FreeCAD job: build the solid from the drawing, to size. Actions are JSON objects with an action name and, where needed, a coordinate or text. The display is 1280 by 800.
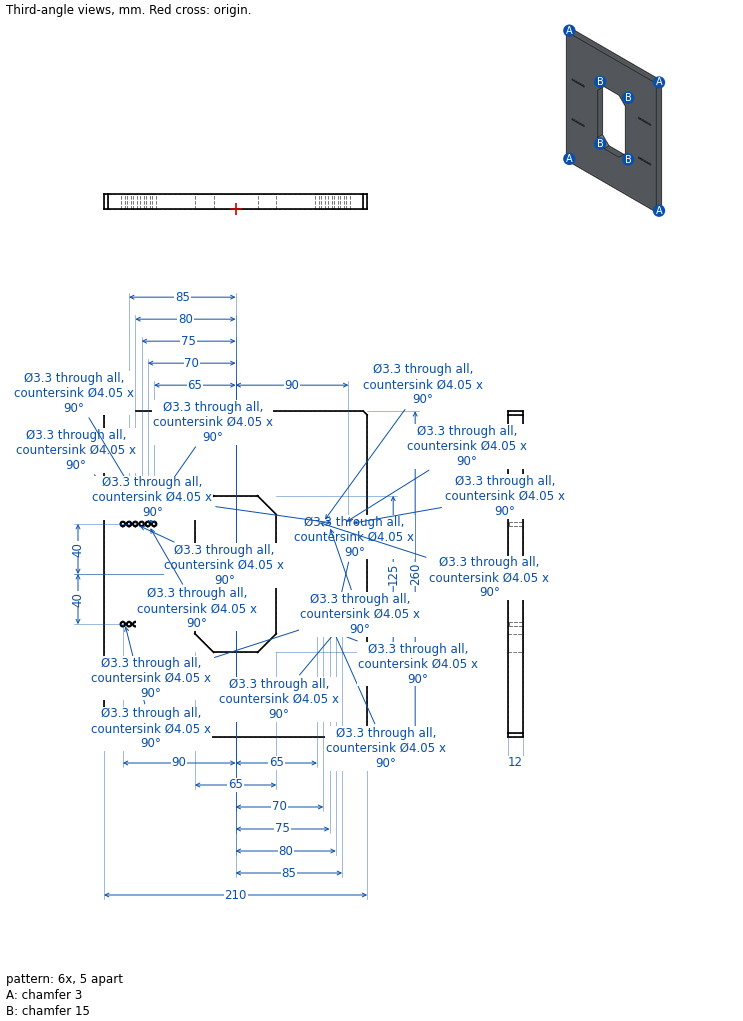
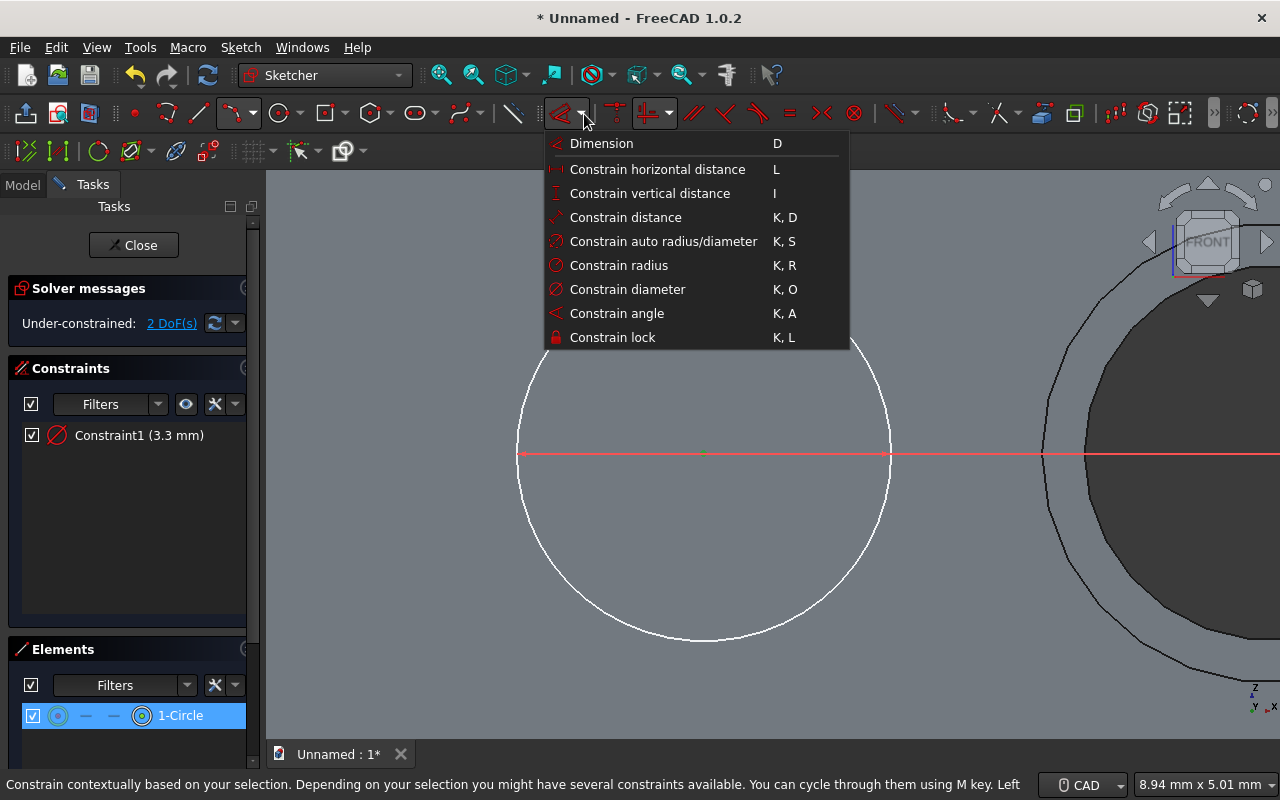
{"action": "left_click", "coordinate": [697, 169]}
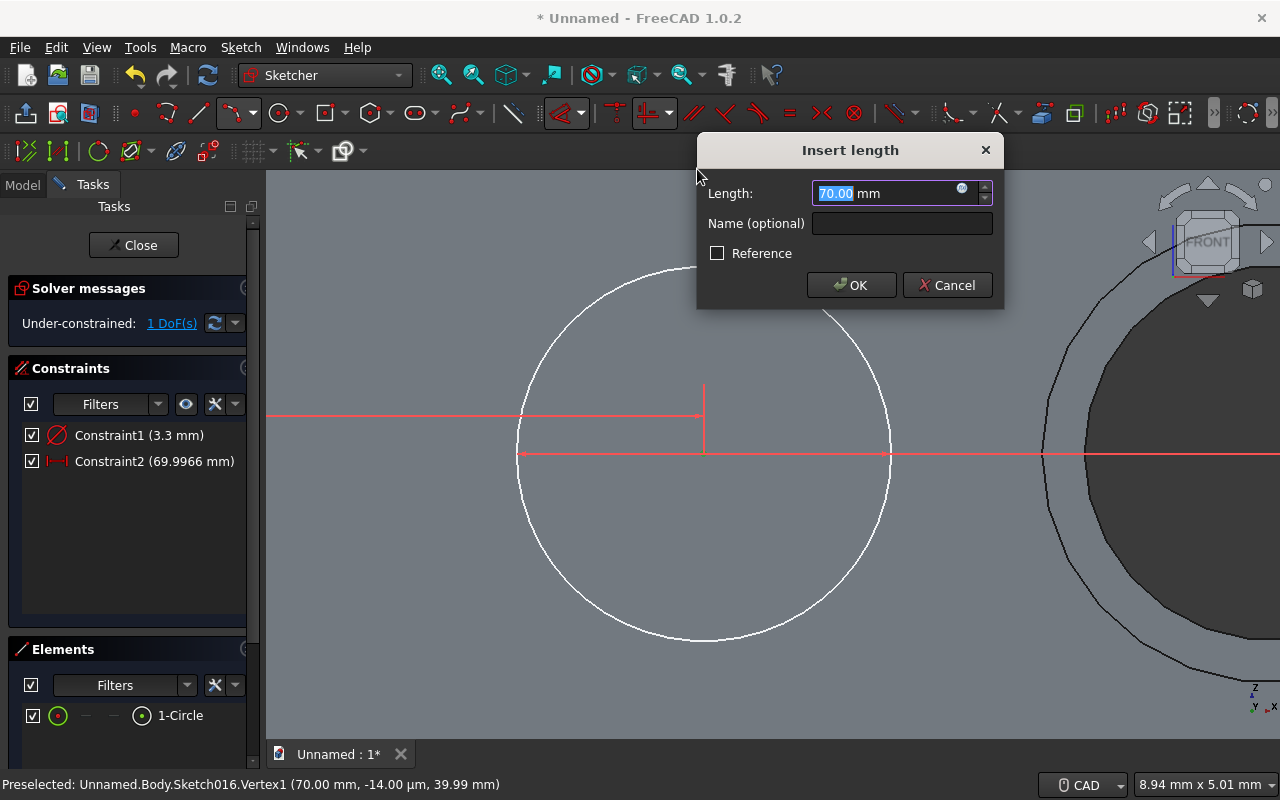
{"action": "type", "text": "70"}
{"action": "key", "text": "Return"}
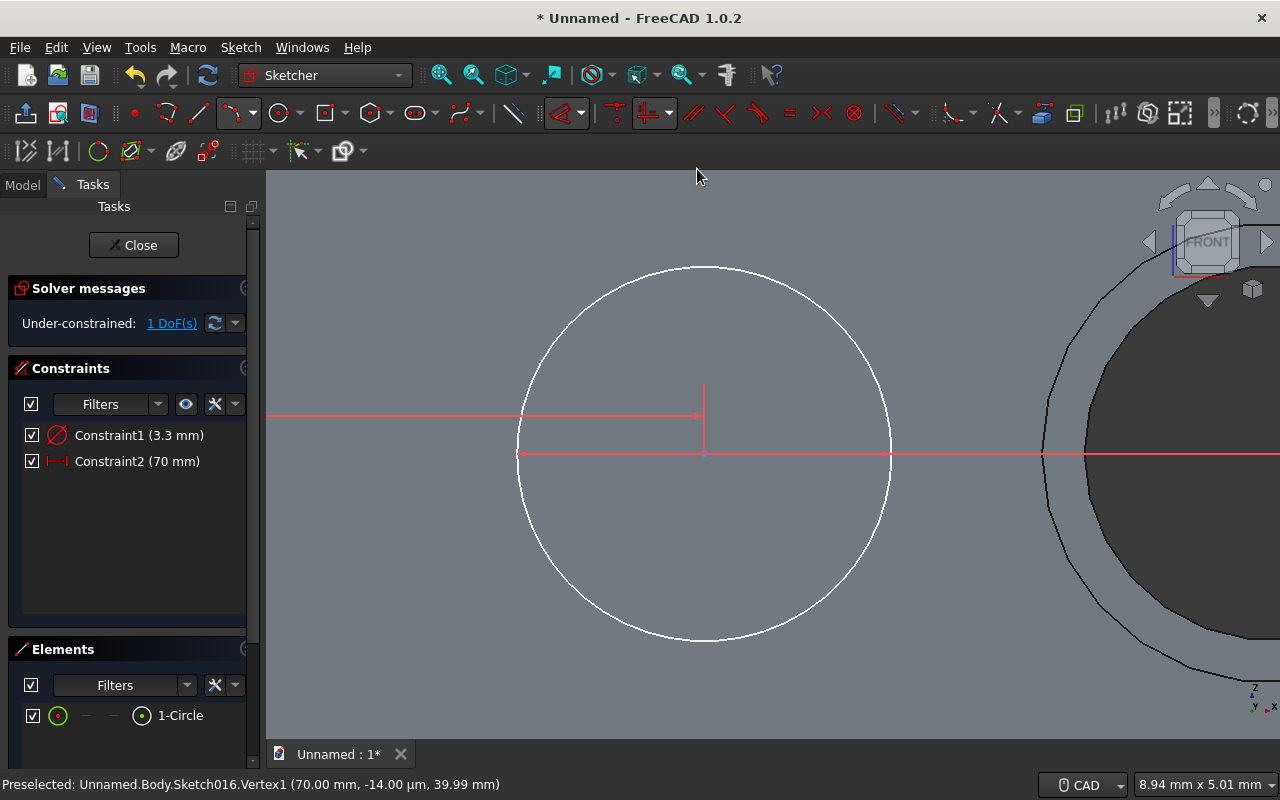
{"action": "left_click", "coordinate": [704, 454]}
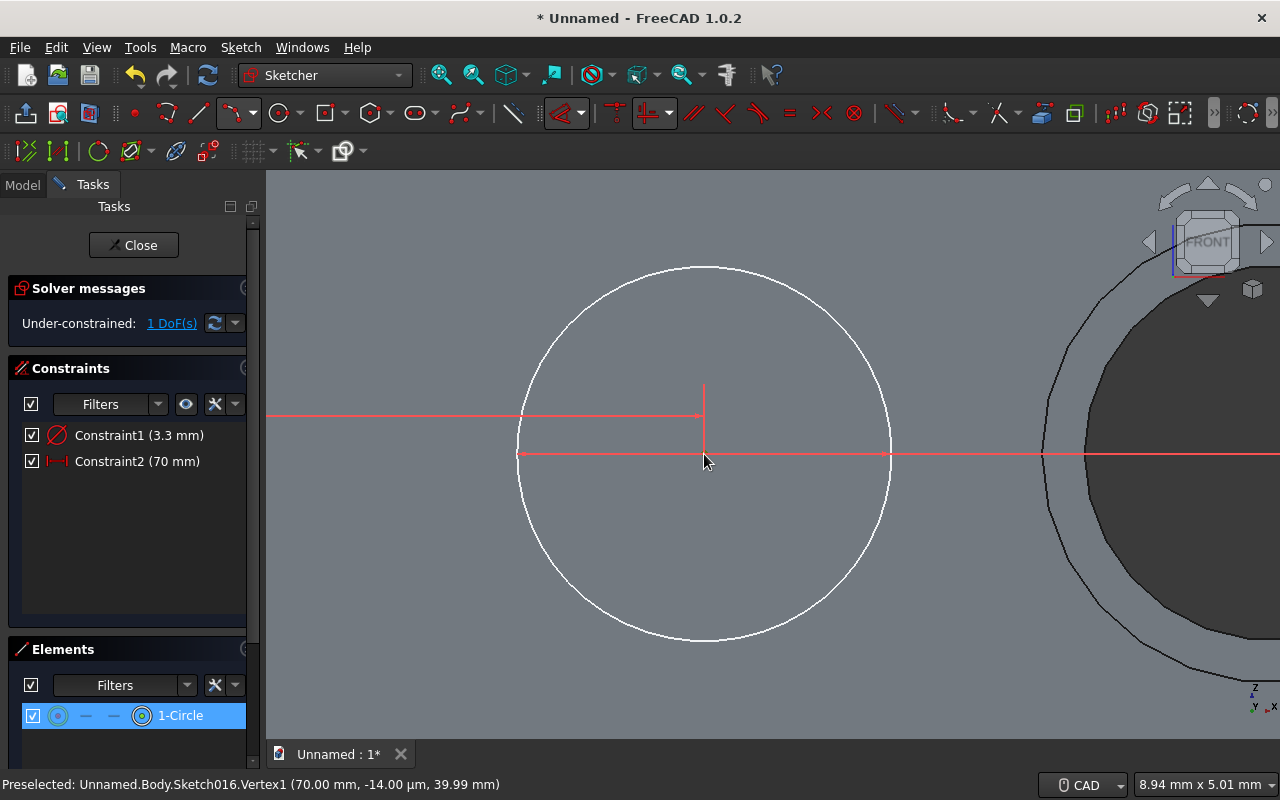
{"action": "left_click", "coordinate": [584, 114]}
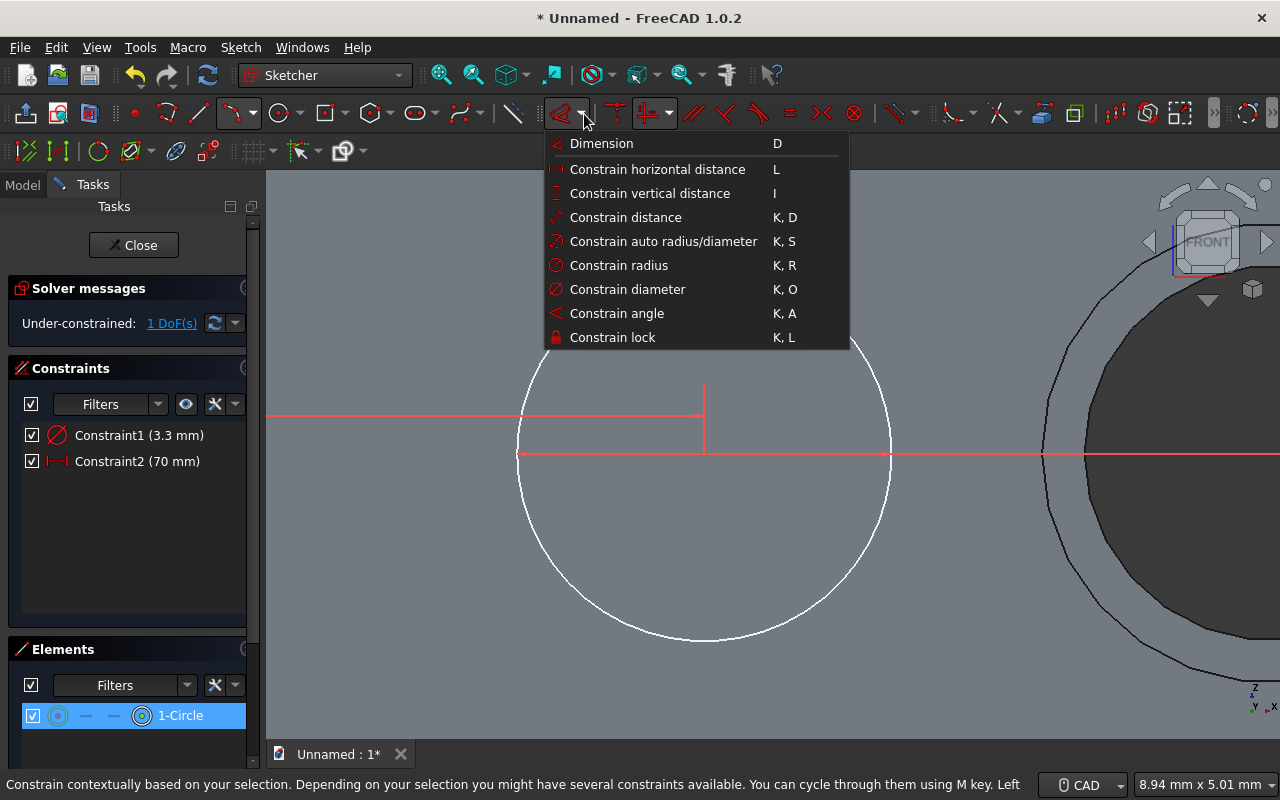
{"action": "left_click", "coordinate": [697, 193]}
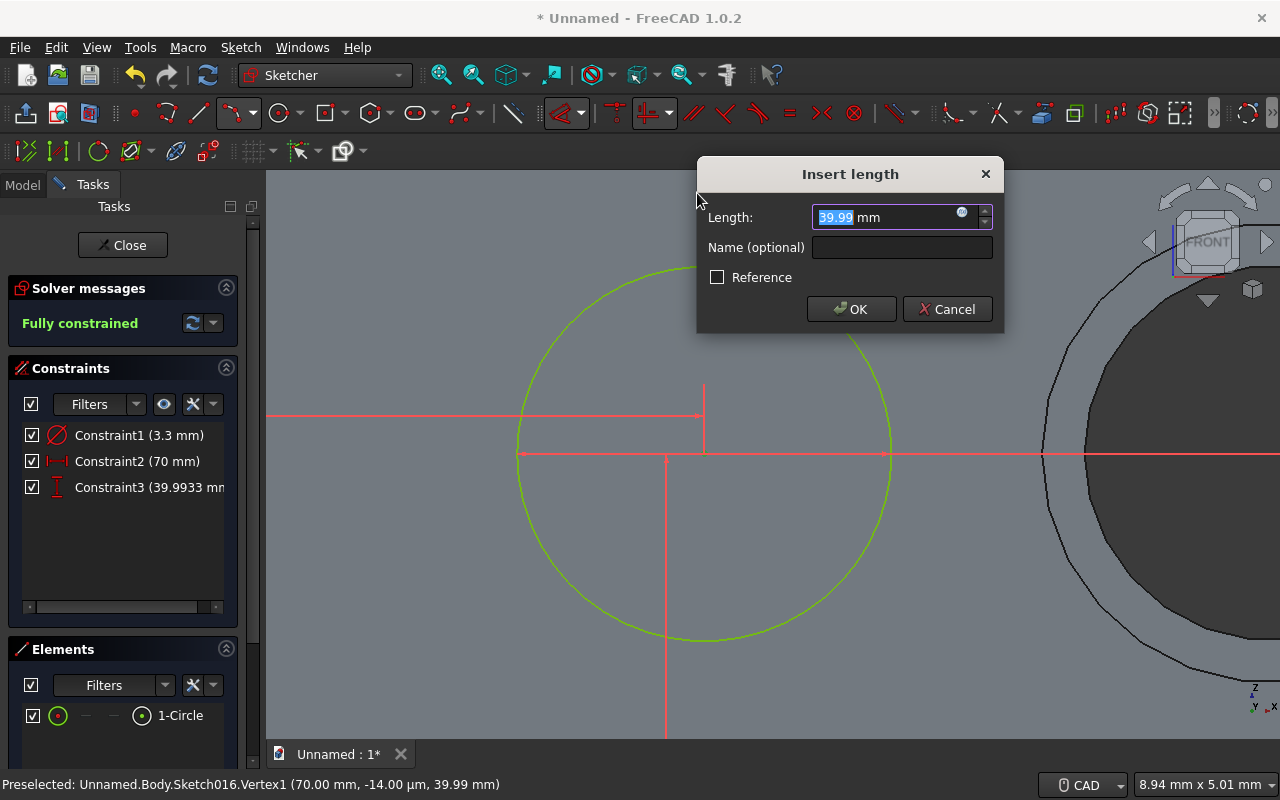
{"action": "type", "text": "40"}
{"action": "key", "text": "Return"}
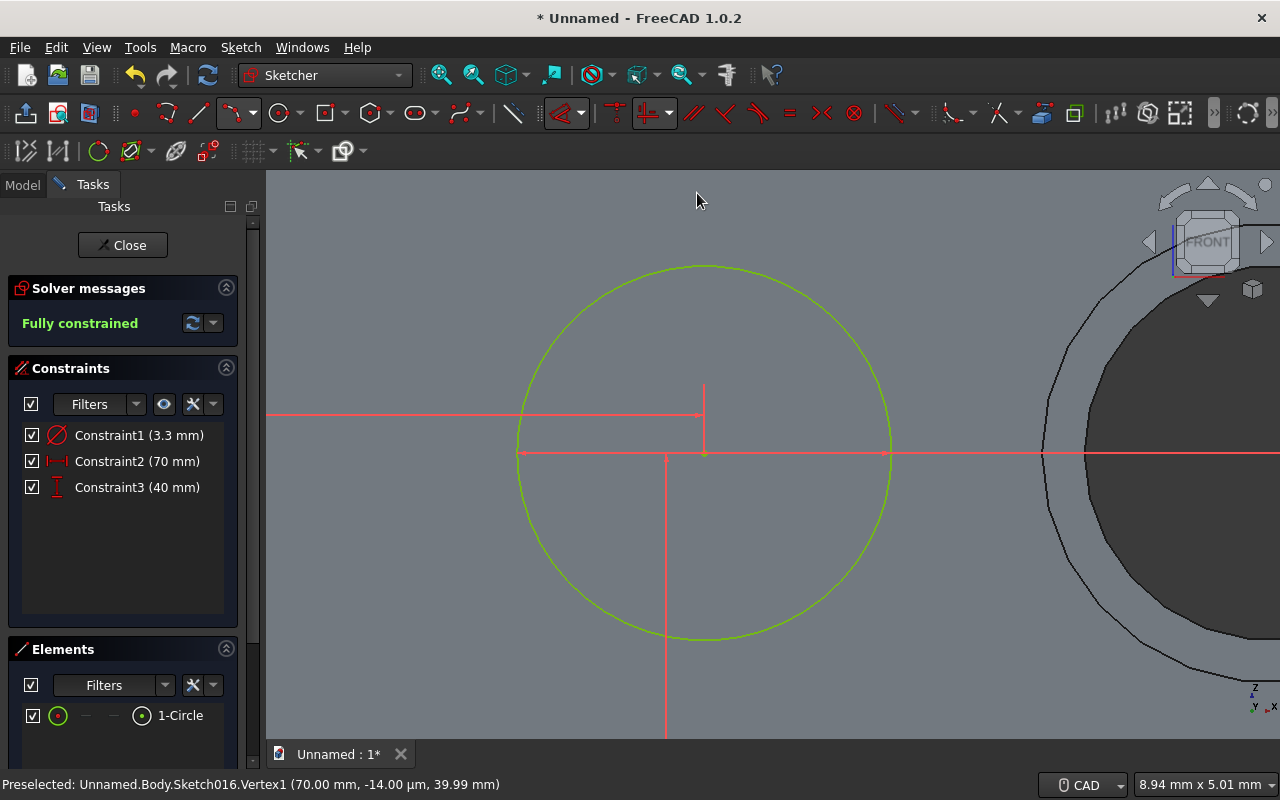
{"action": "left_click", "coordinate": [123, 245]}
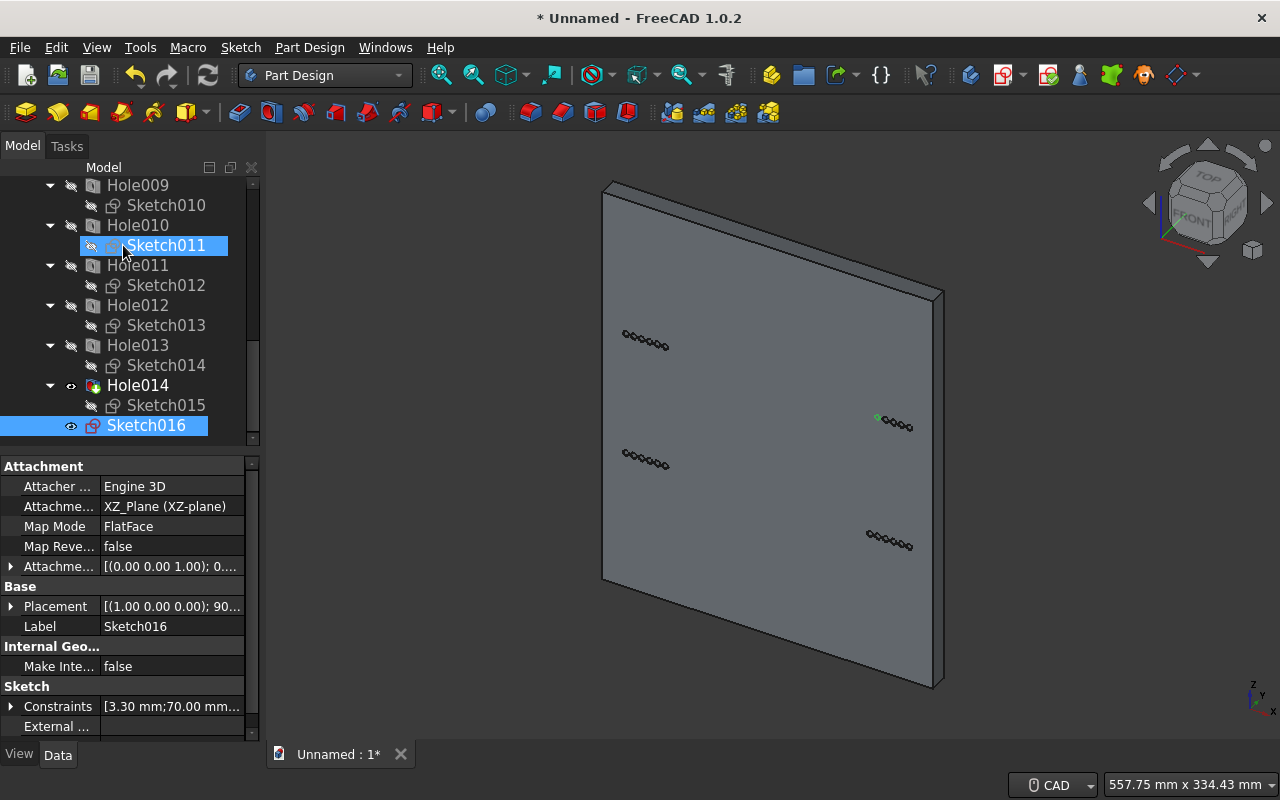
{"action": "left_click", "coordinate": [272, 112]}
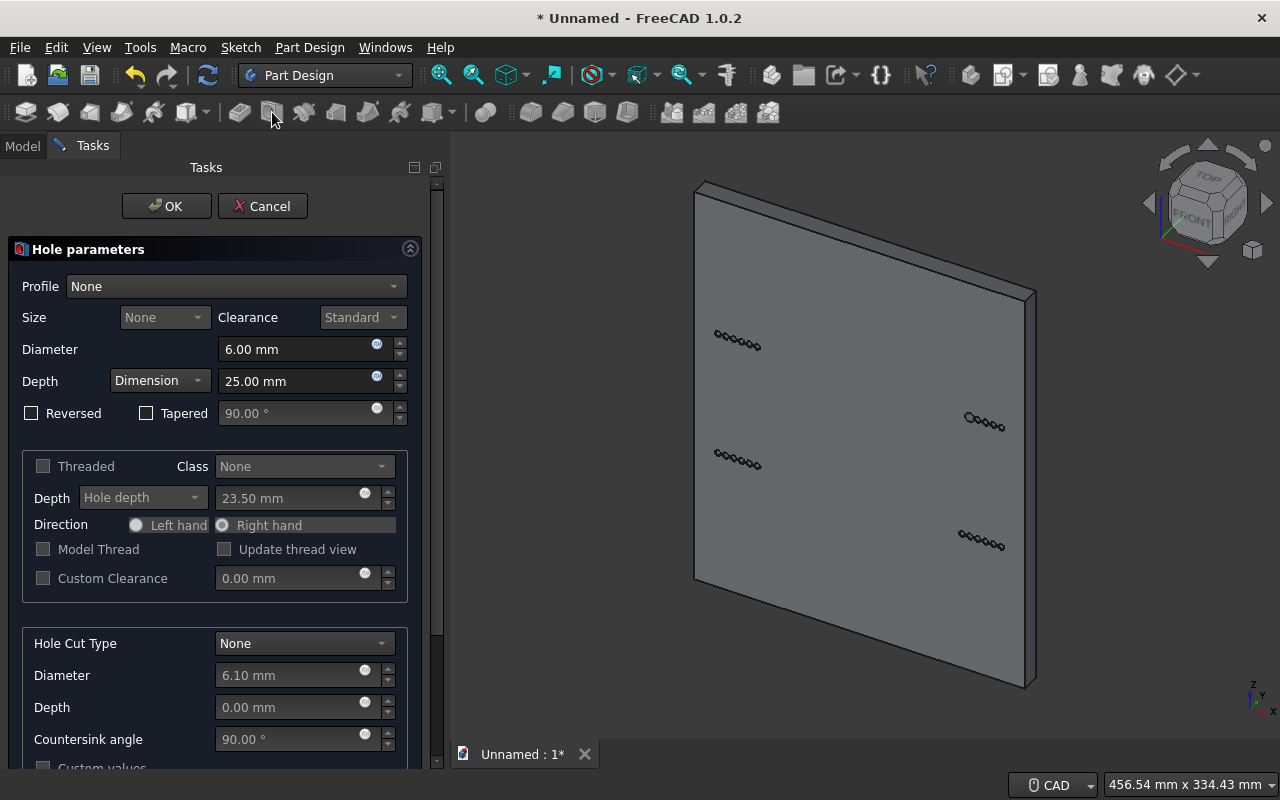
{"action": "triple_click", "coordinate": [305, 349]}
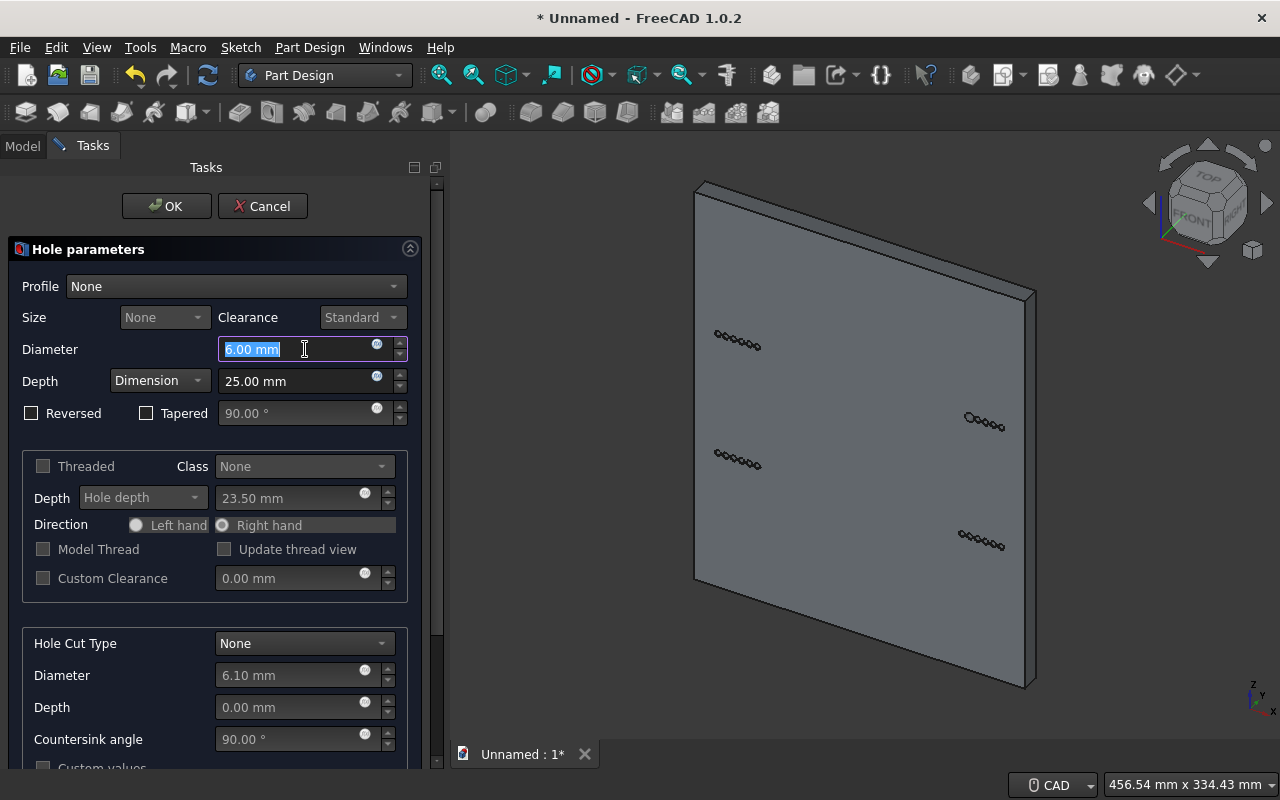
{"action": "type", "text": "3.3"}
{"action": "key", "text": "Tab"}